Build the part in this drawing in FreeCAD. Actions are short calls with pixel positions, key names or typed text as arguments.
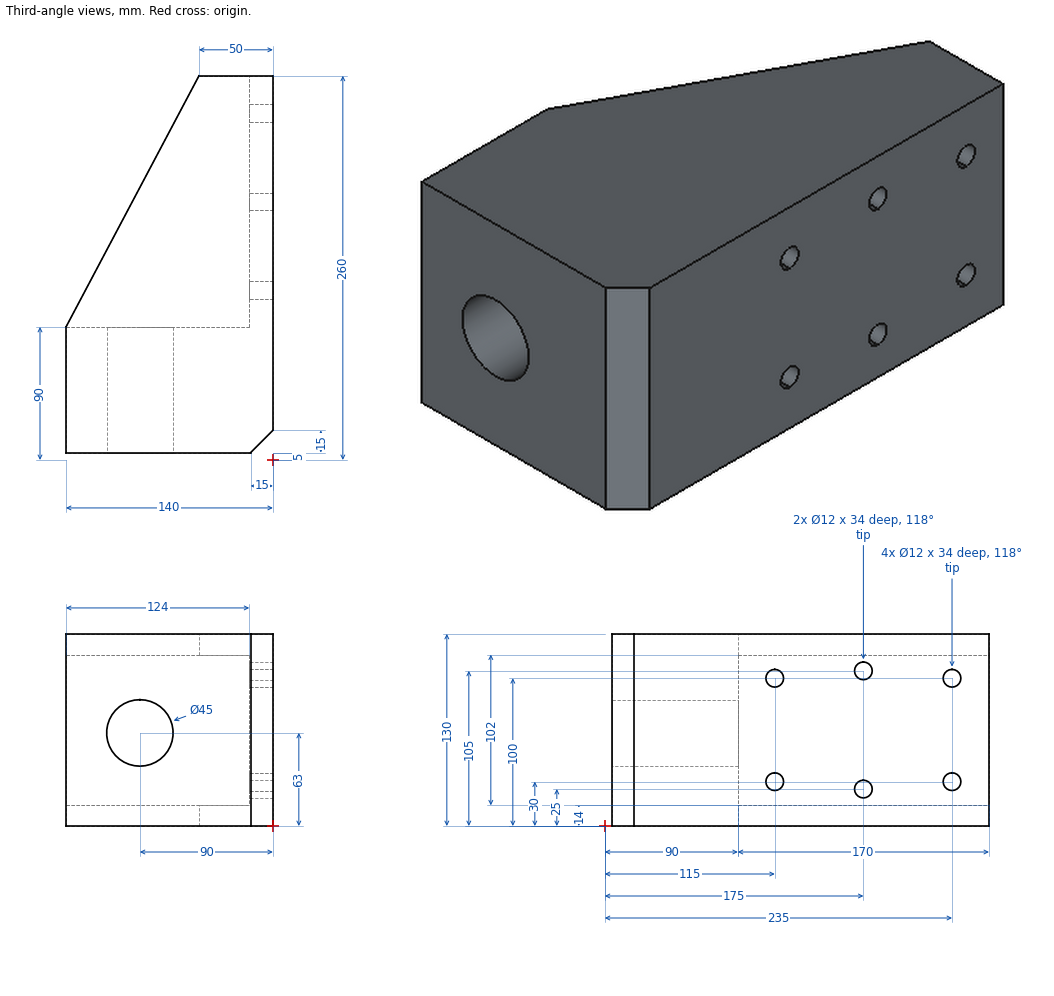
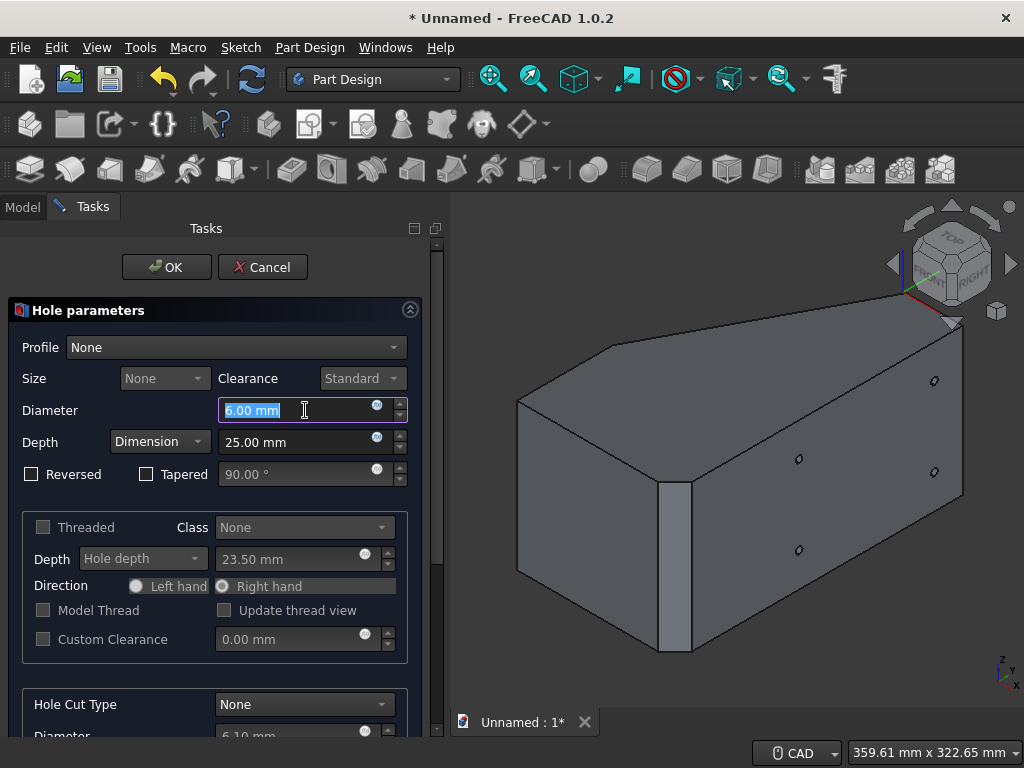
text(12)
key(Tab)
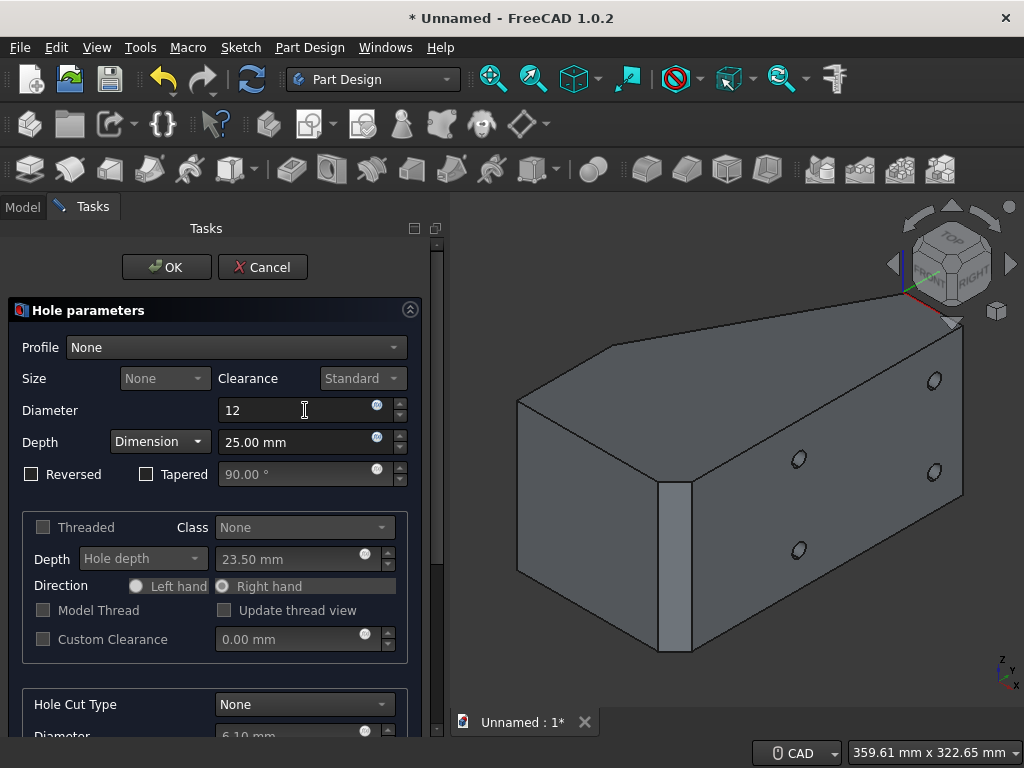
triple_click(305, 442)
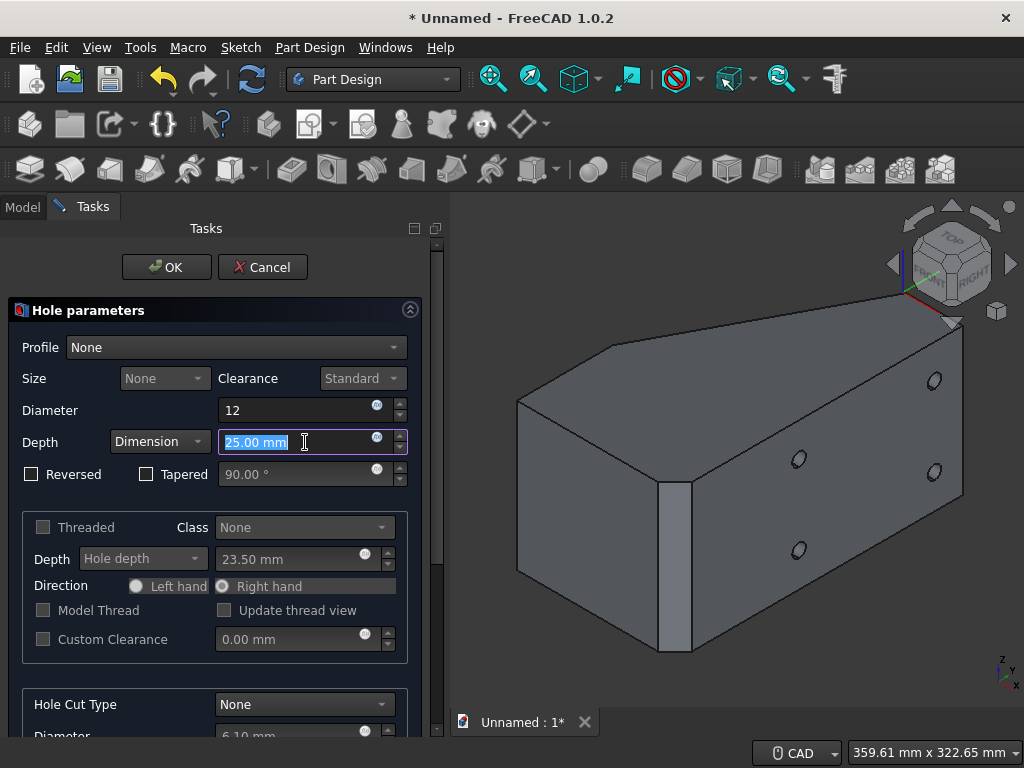
text(34)
key(Tab)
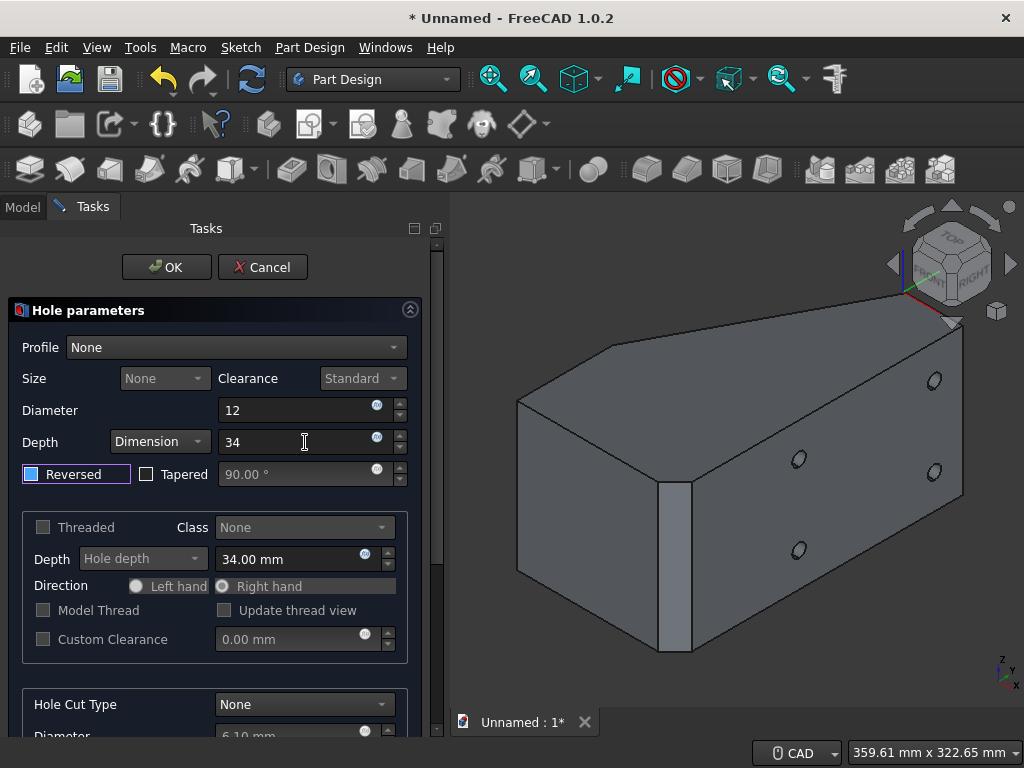
click(167, 267)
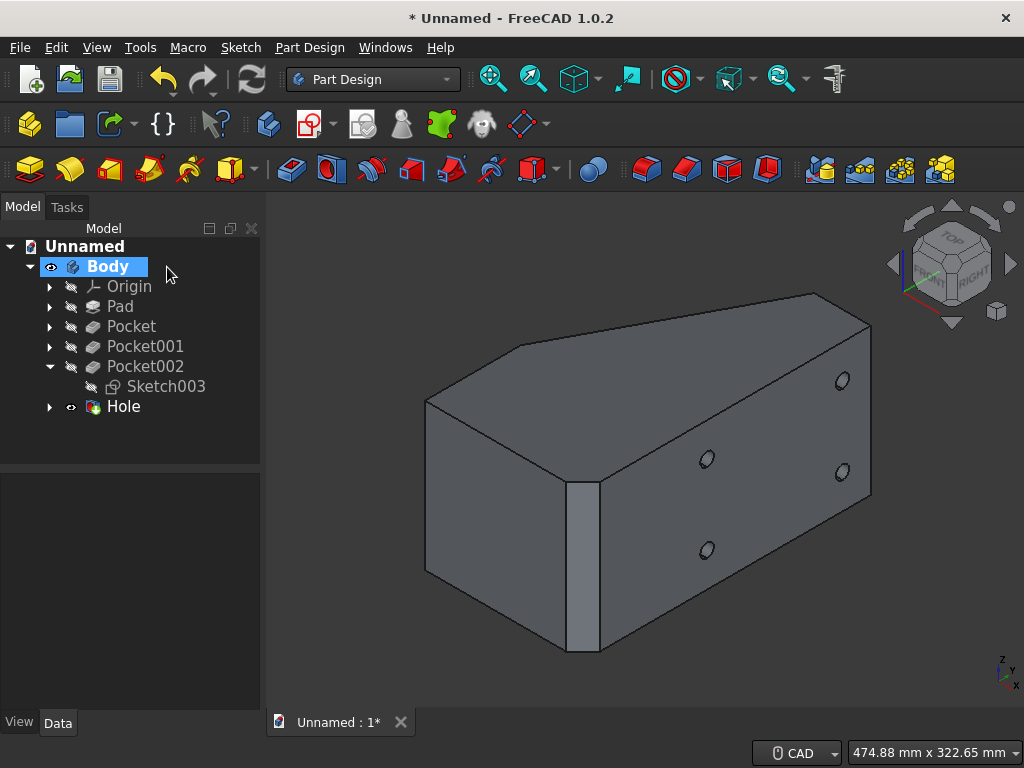
click(310, 124)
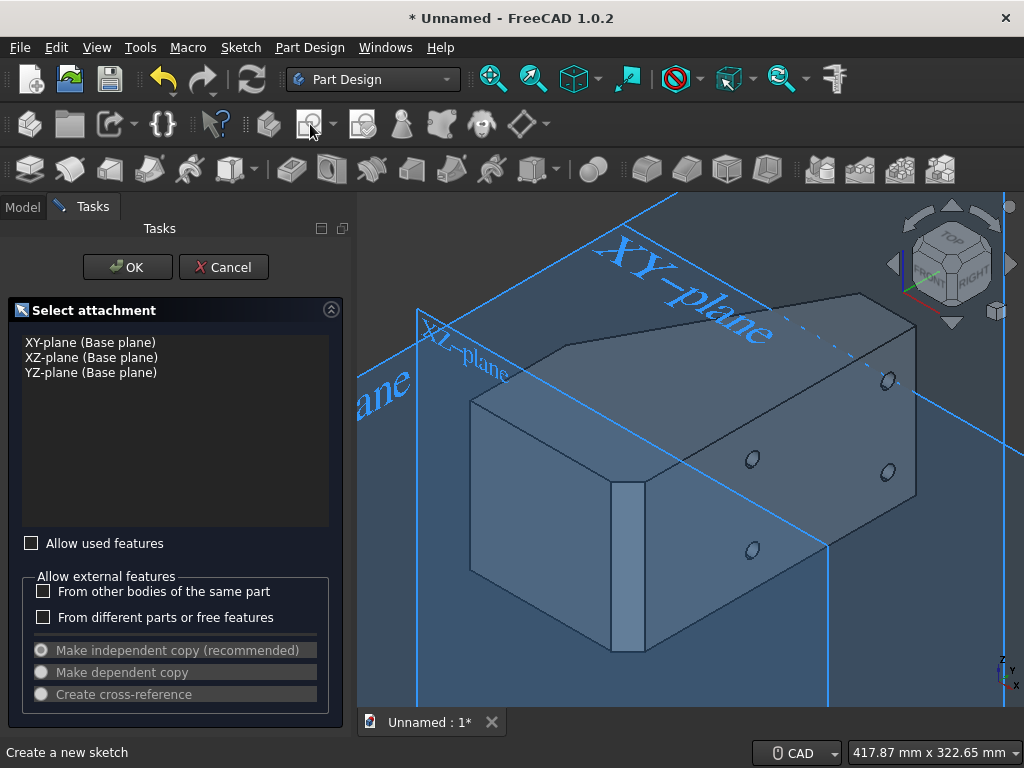
click(82, 372)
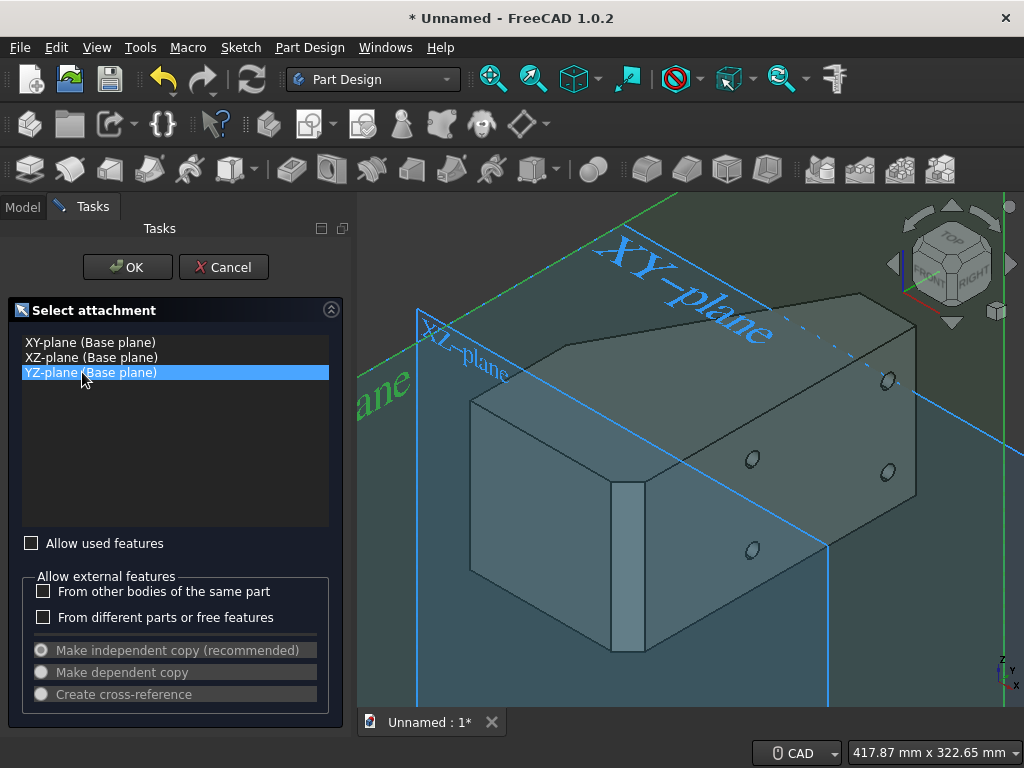
click(128, 267)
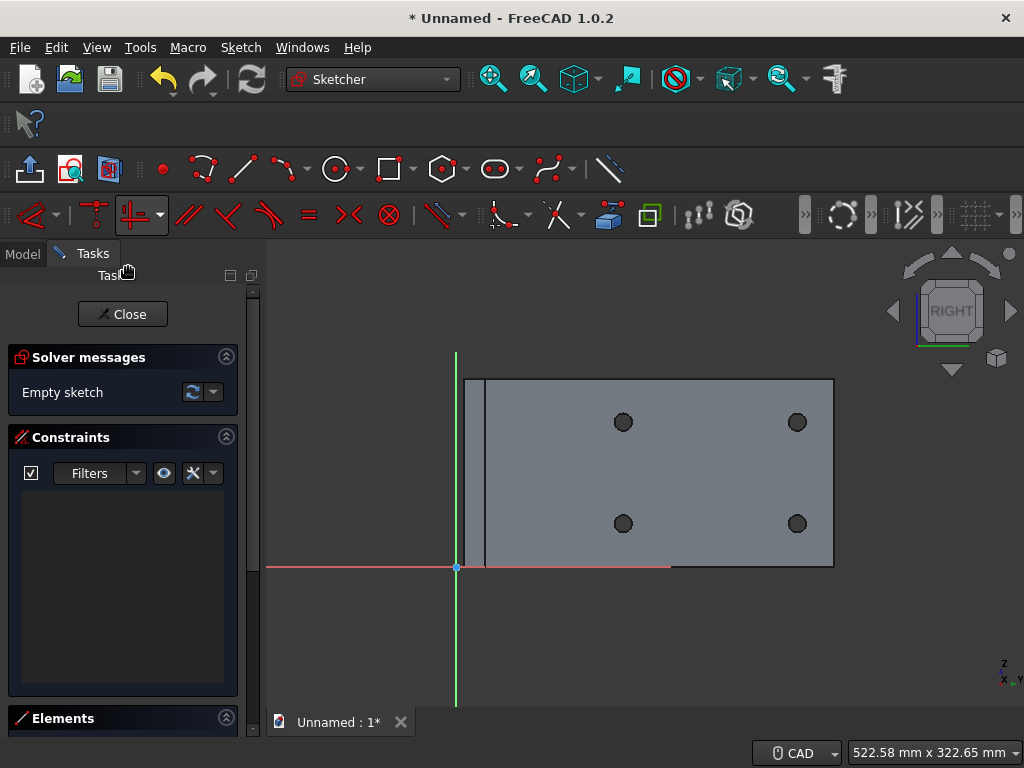
scroll(610, 515, up, 2)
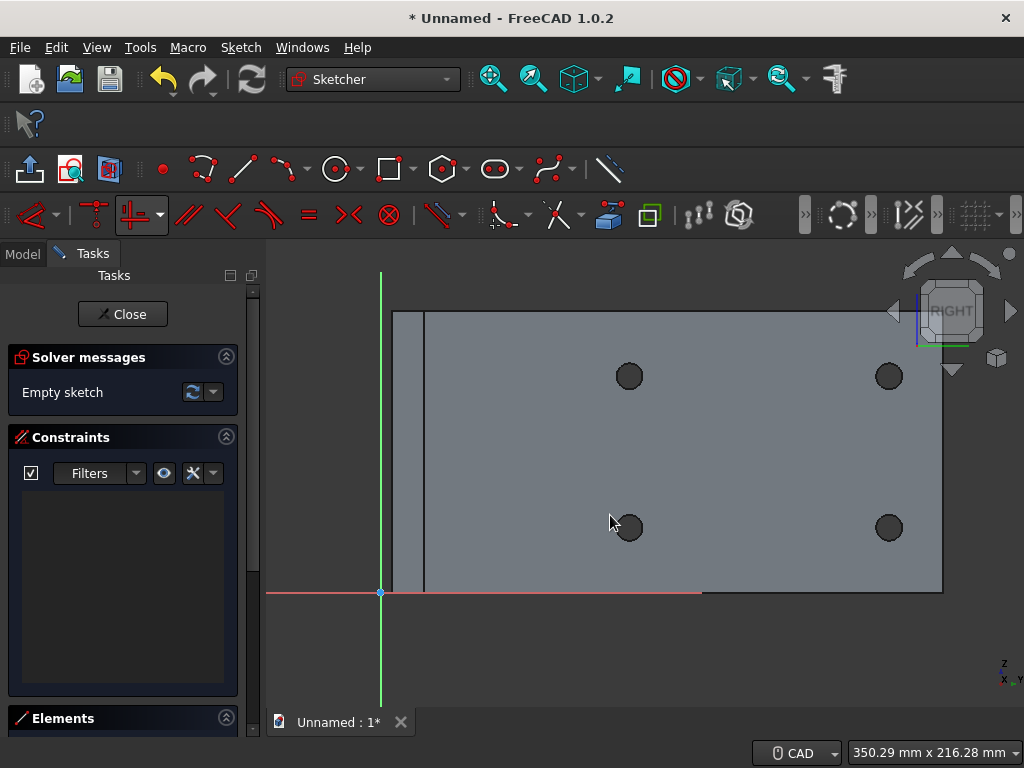
click(336, 170)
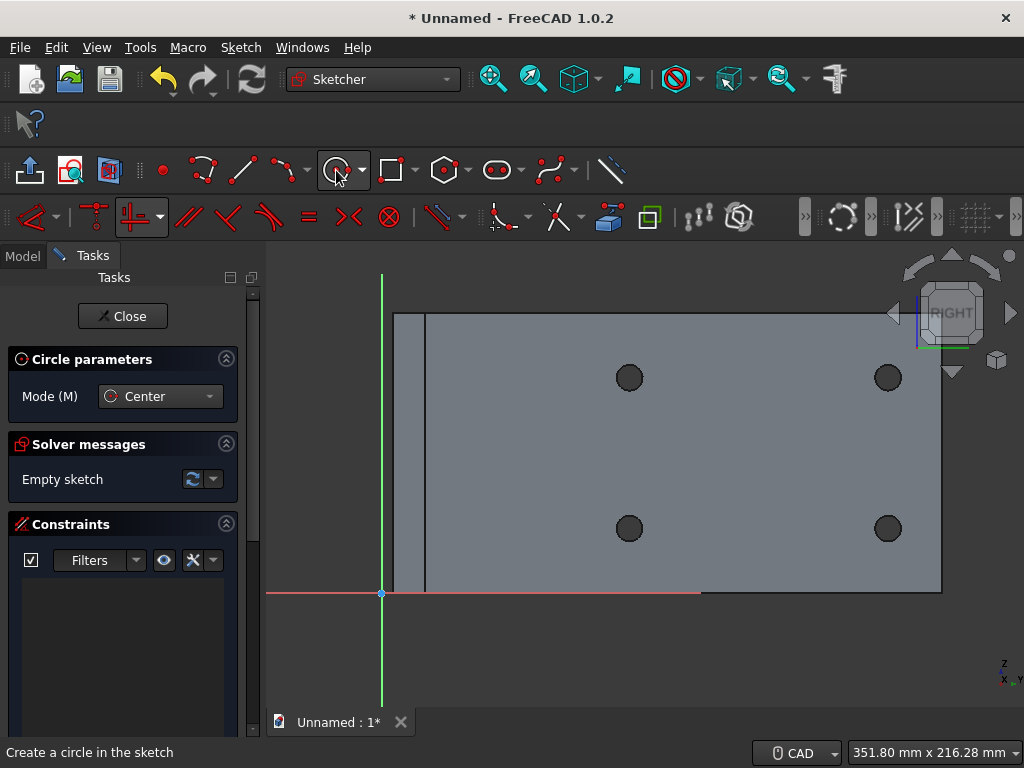
scroll(759, 367, up, 3)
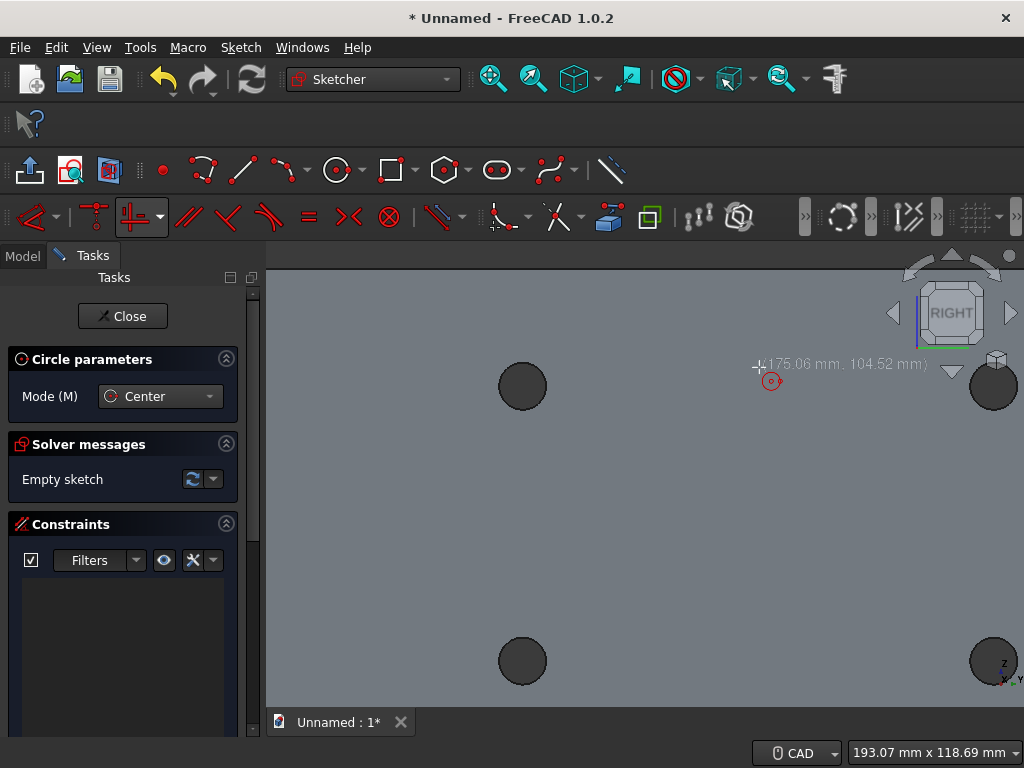
click(758, 367)
move(775, 350)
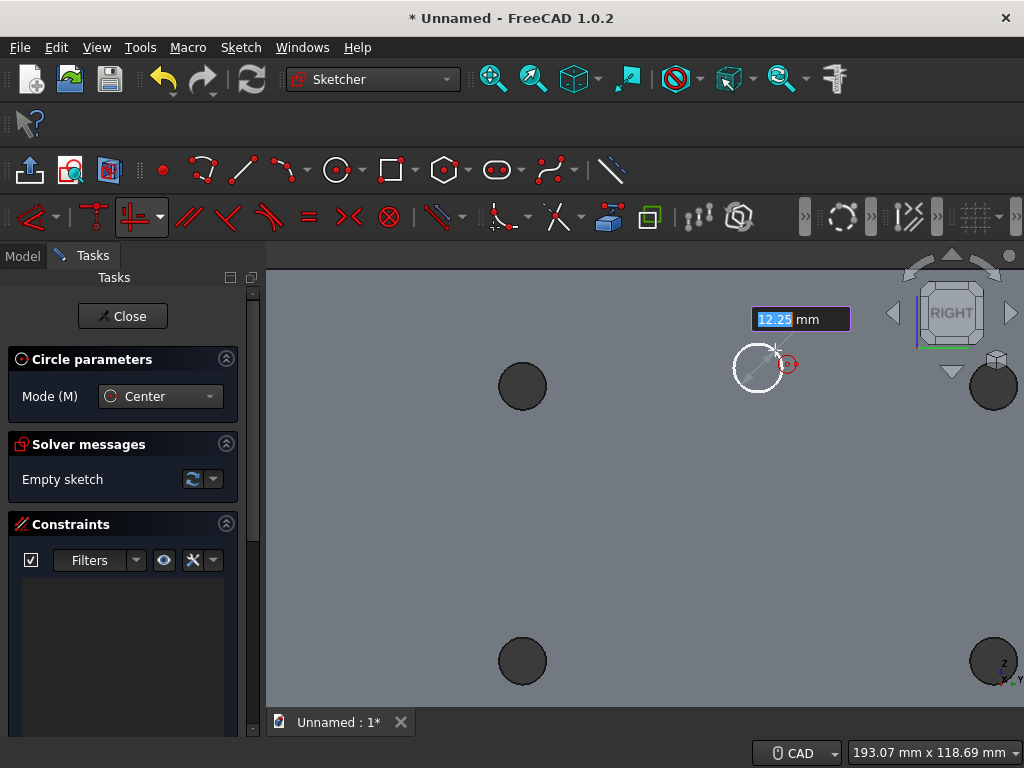
text(12)
key(Return)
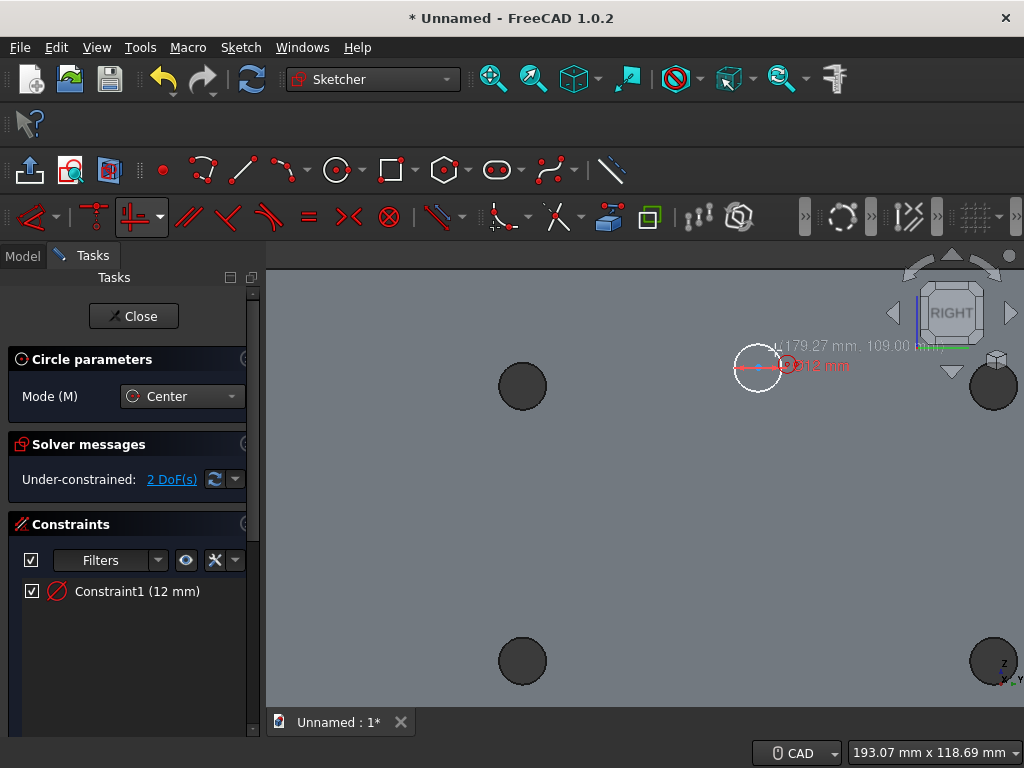
scroll(759, 368, down, 3)